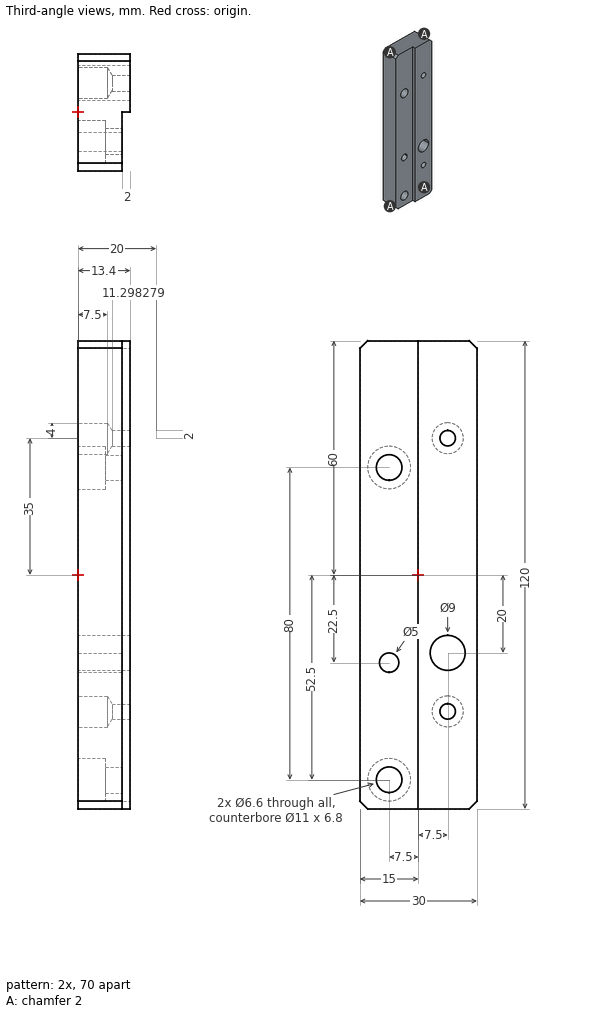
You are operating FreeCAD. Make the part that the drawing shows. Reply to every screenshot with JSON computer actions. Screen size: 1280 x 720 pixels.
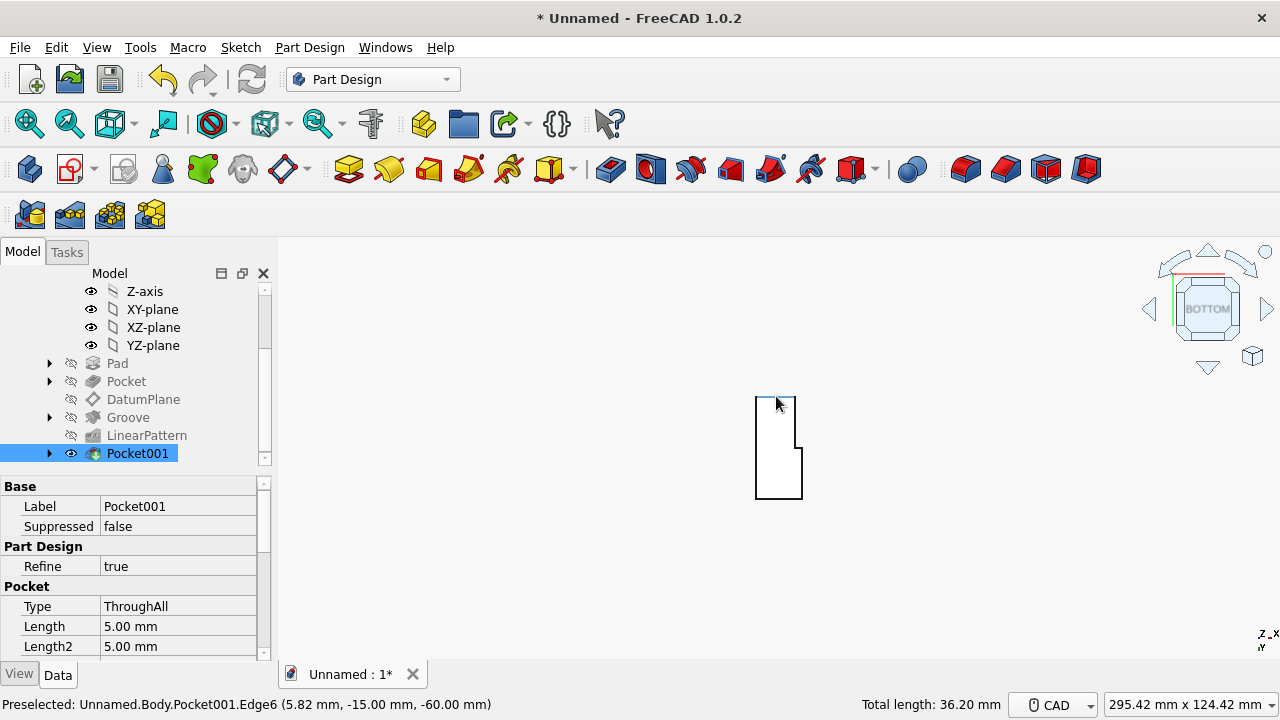
{"action": "left_click", "coordinate": [779, 498], "text": "ctrl"}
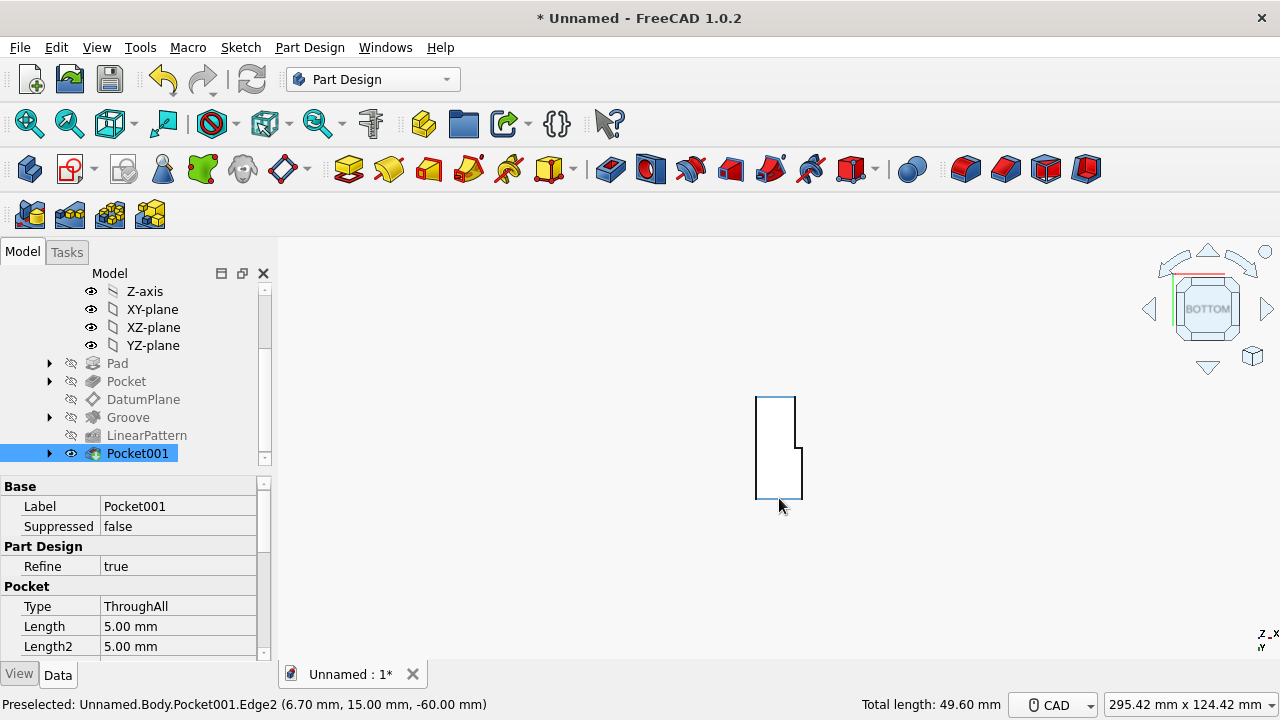
{"action": "left_click", "coordinate": [1006, 170]}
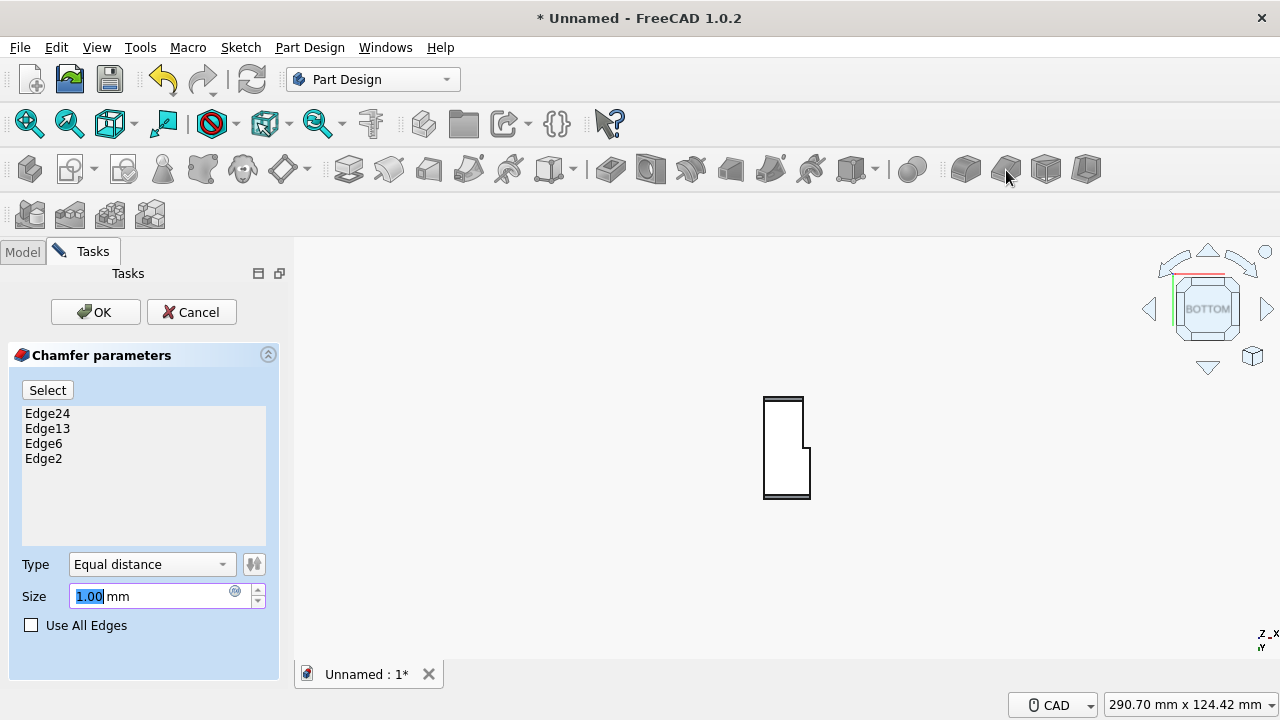
{"action": "type", "text": "2"}
{"action": "key", "text": "Tab"}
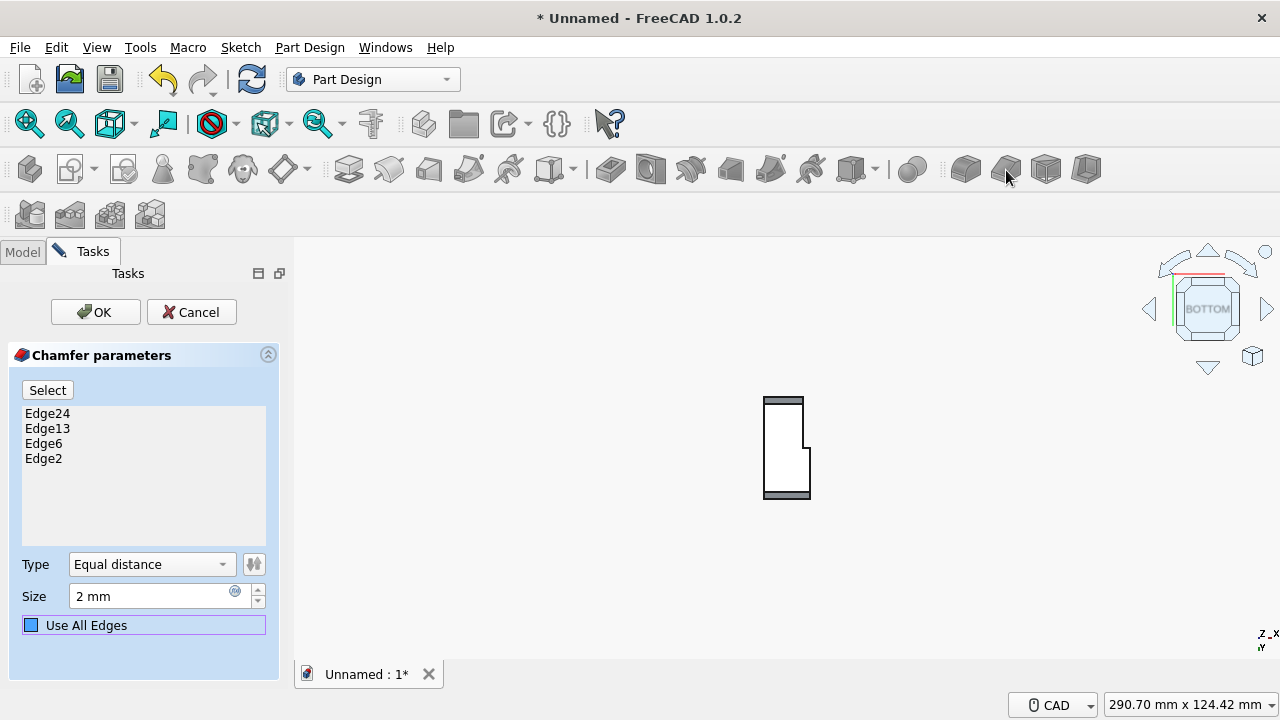
{"action": "left_click", "coordinate": [96, 312]}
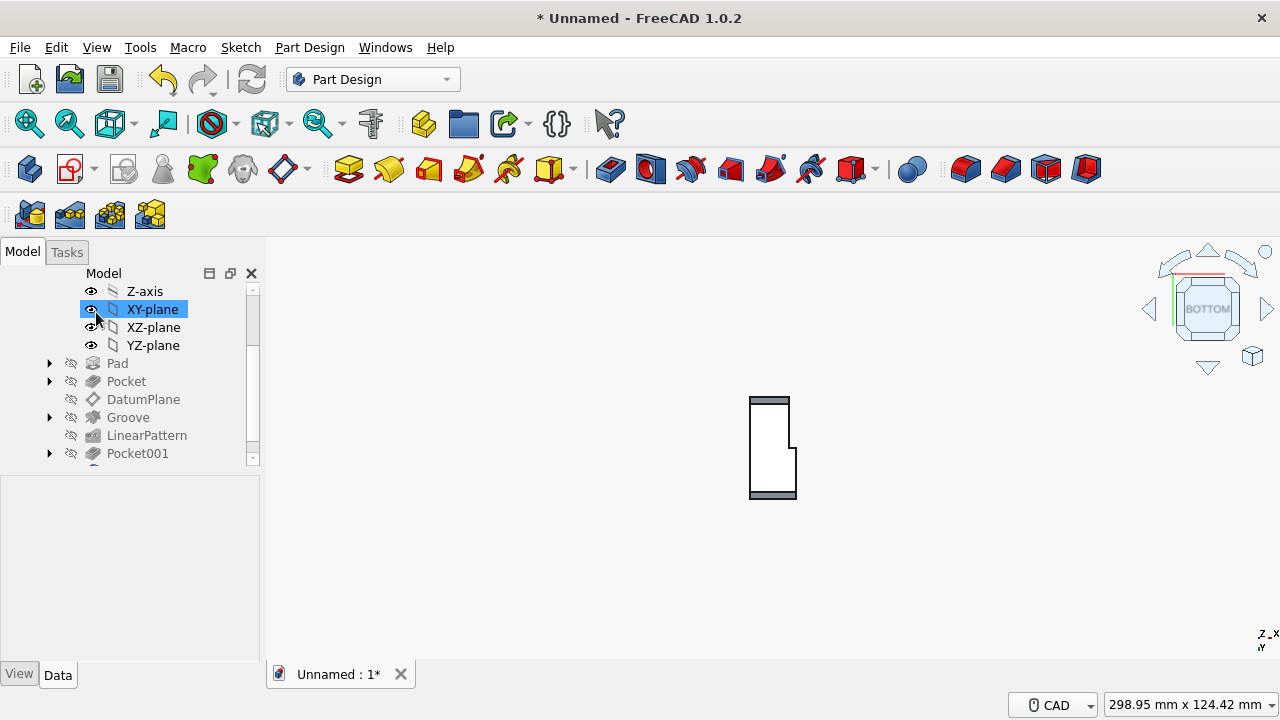
{"action": "left_click", "coordinate": [30, 124]}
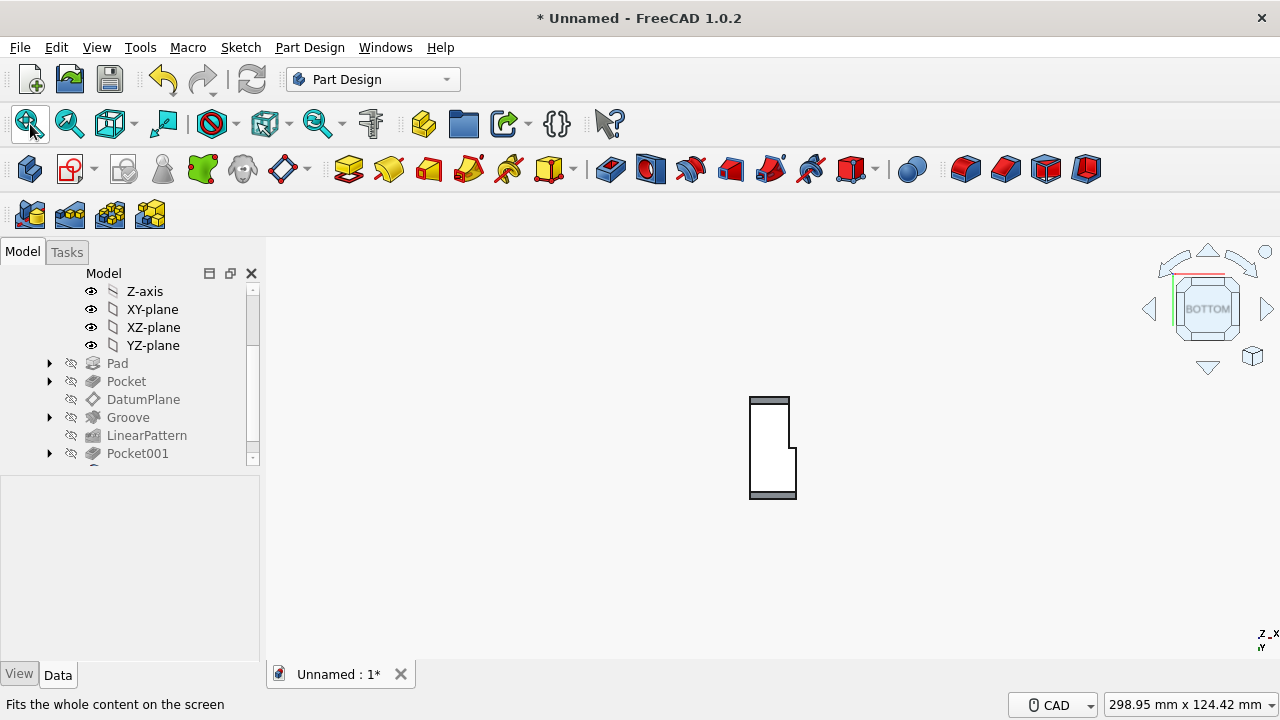
{"action": "left_click", "coordinate": [70, 170]}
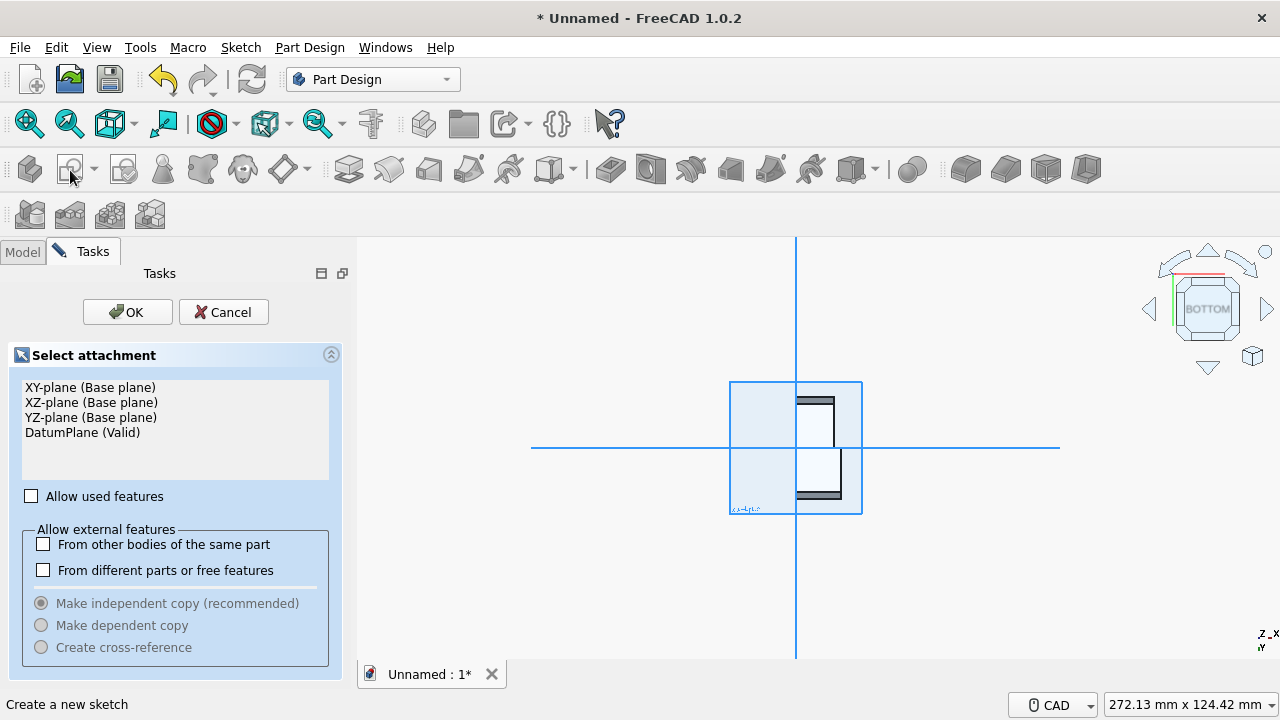
{"action": "left_click", "coordinate": [82, 418]}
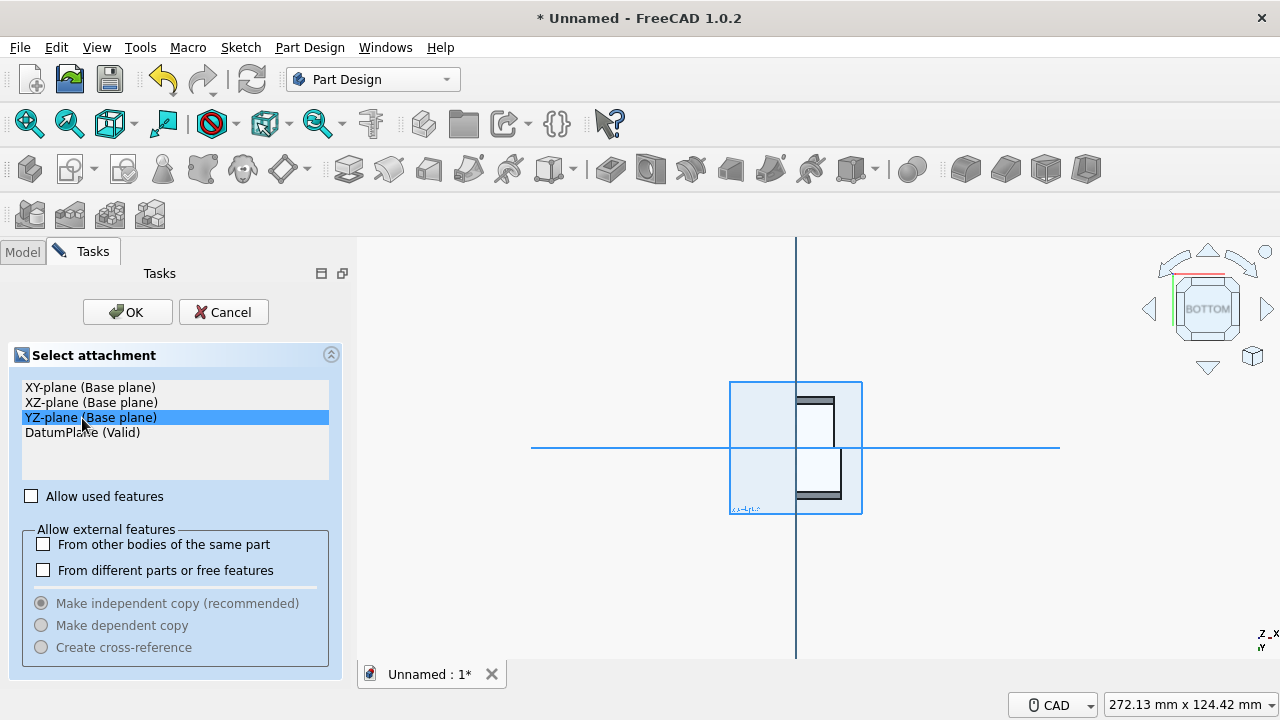
{"action": "left_click", "coordinate": [128, 312]}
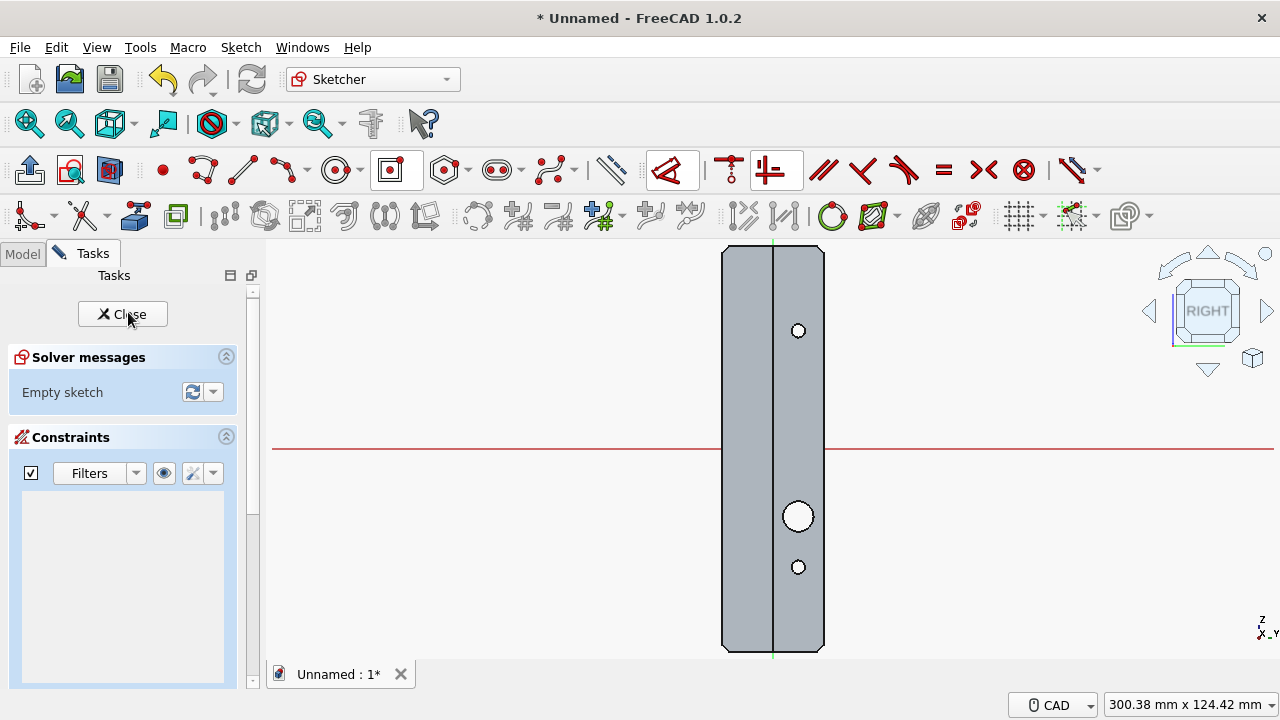
{"action": "left_click", "coordinate": [110, 170]}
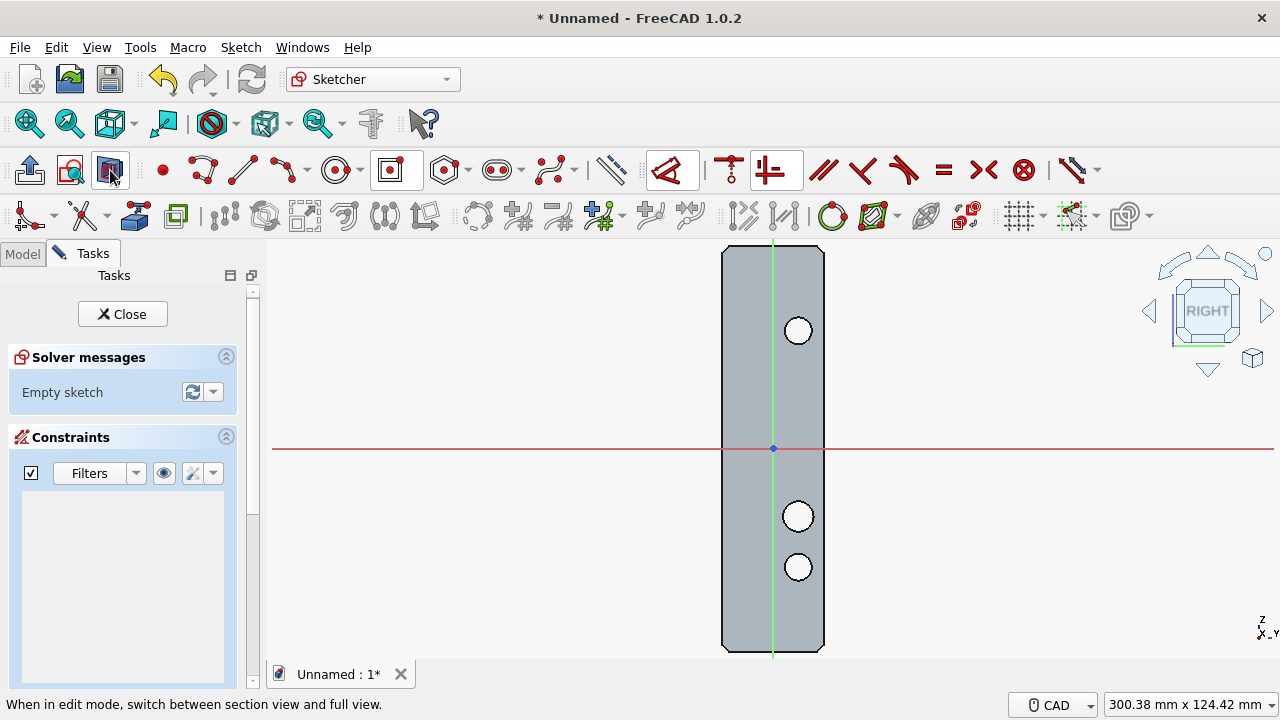
{"action": "scroll", "coordinate": [477, 267], "scroll_direction": "down", "scroll_amount": 1}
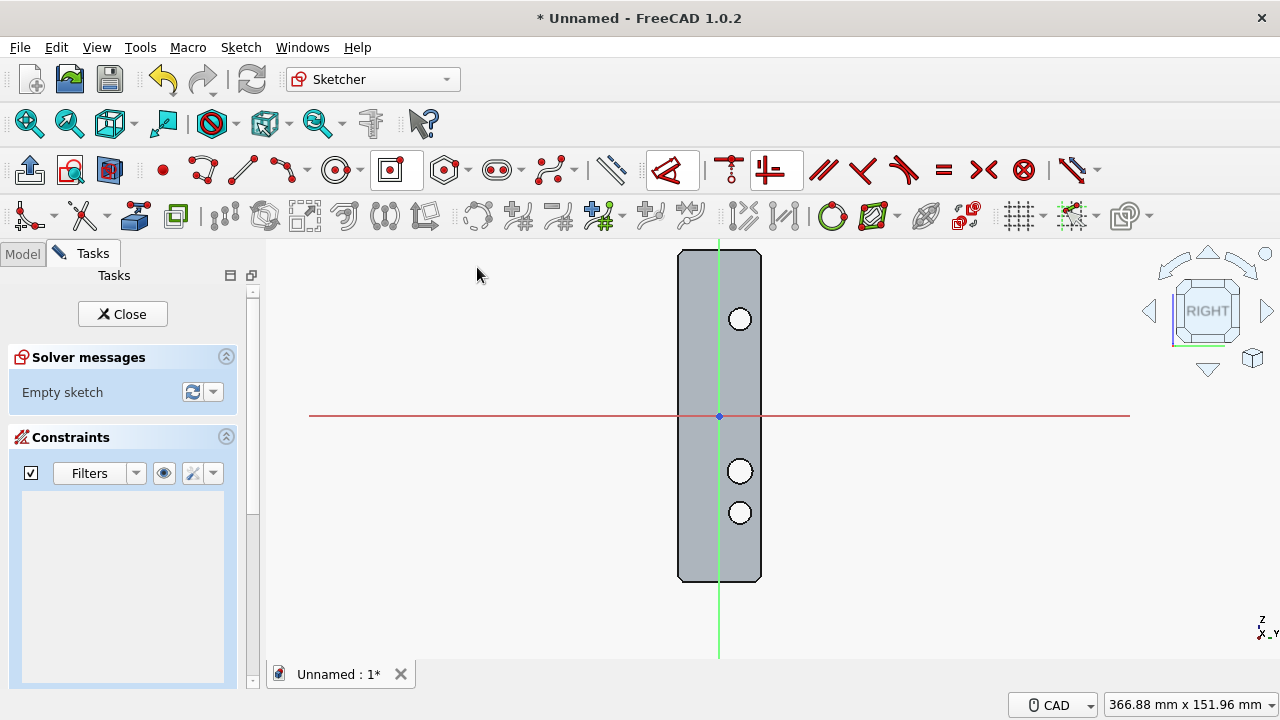
{"action": "left_click", "coordinate": [336, 170]}